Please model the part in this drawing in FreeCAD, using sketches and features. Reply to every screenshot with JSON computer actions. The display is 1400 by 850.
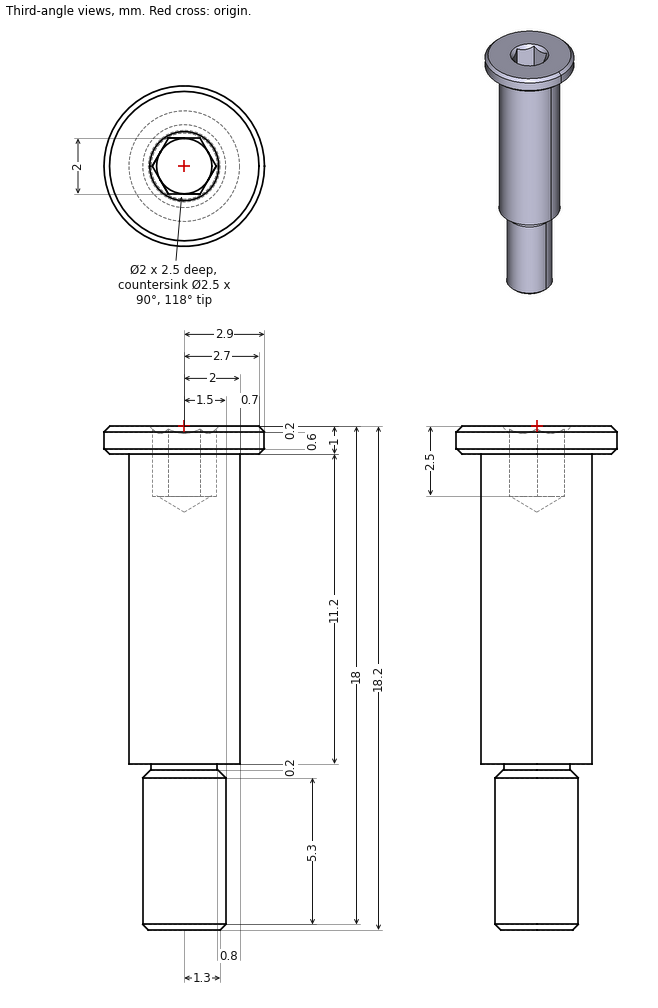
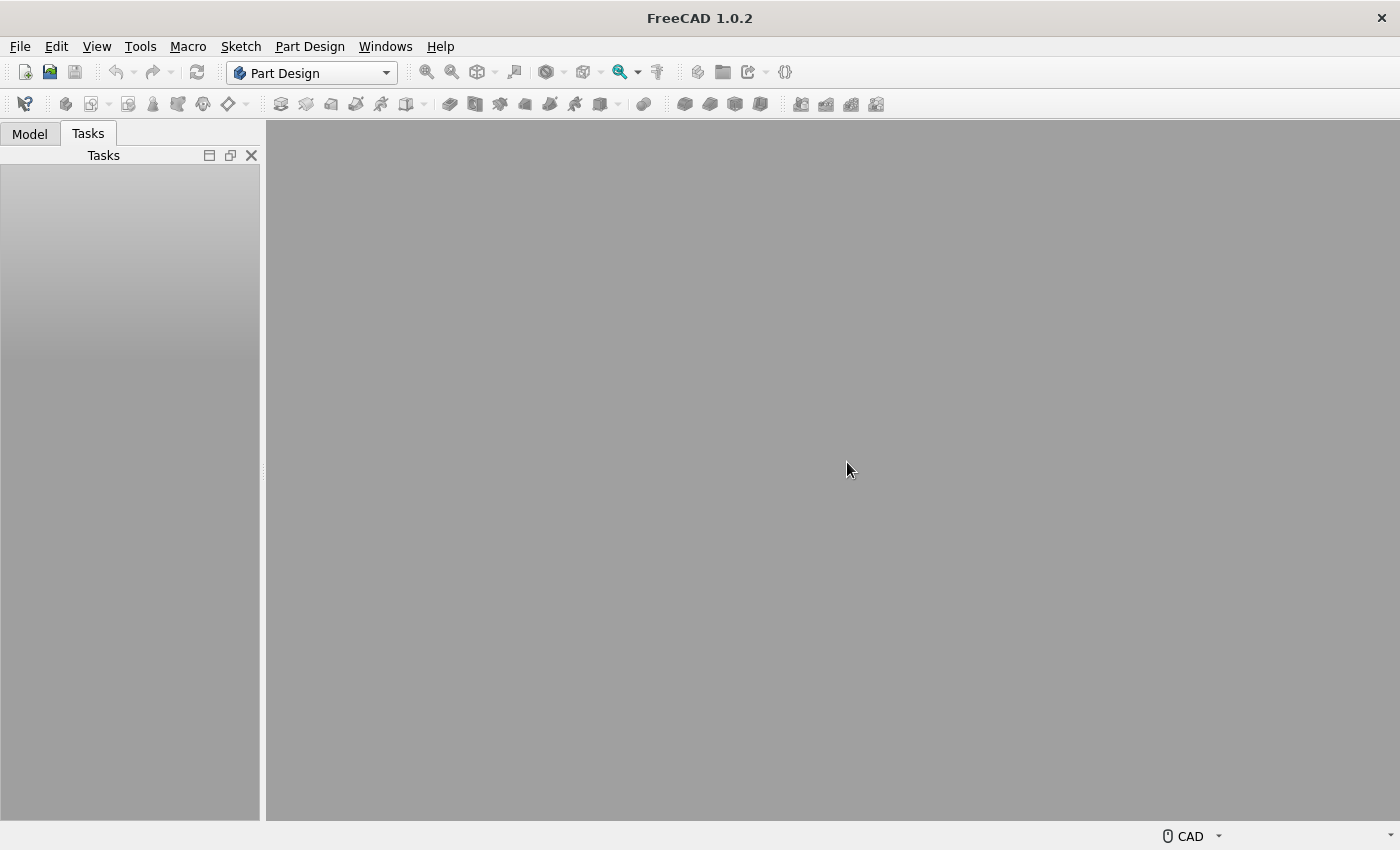
{"action": "left_click", "coordinate": [25, 72]}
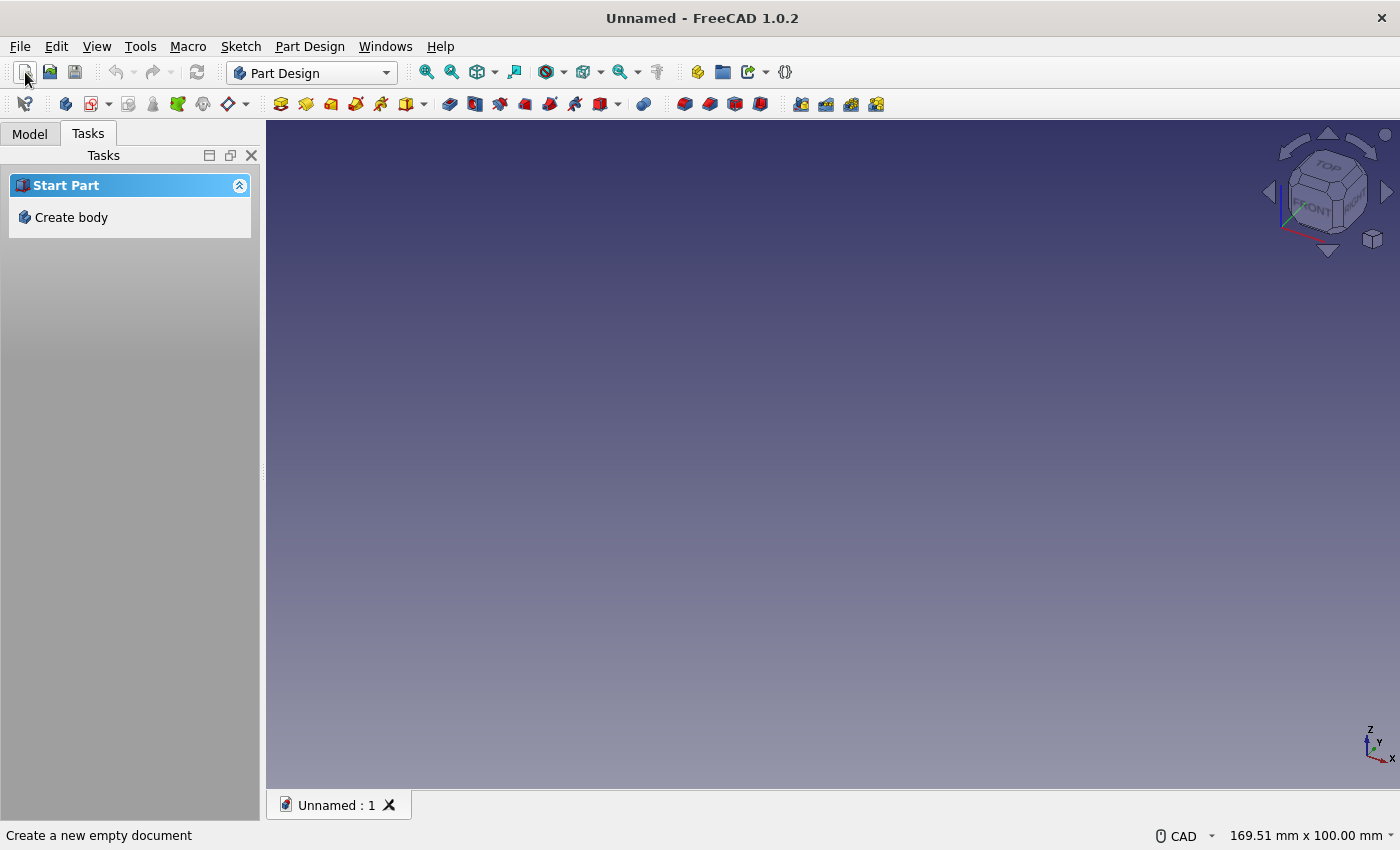
{"action": "left_click", "coordinate": [90, 104]}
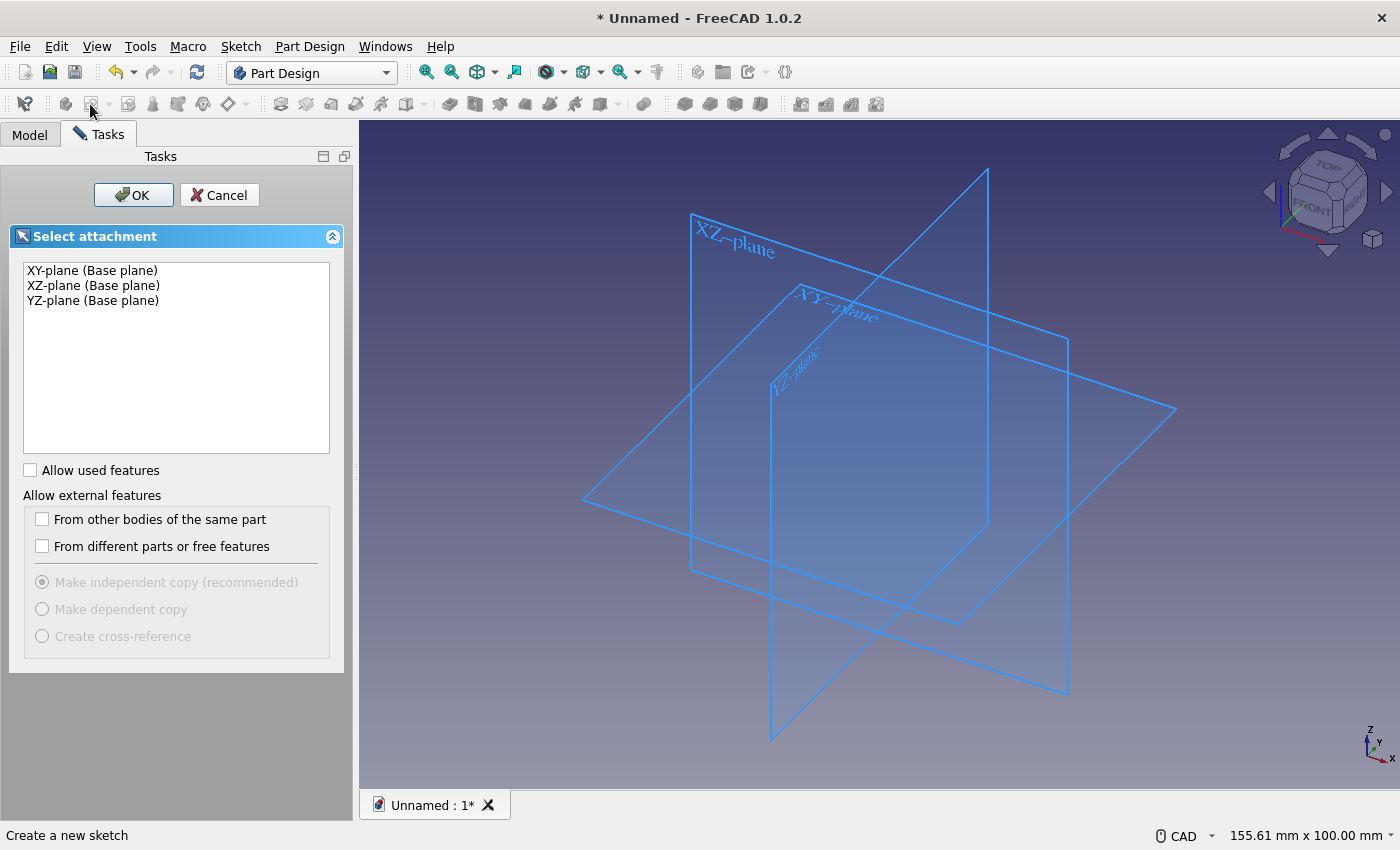
{"action": "left_click", "coordinate": [84, 286]}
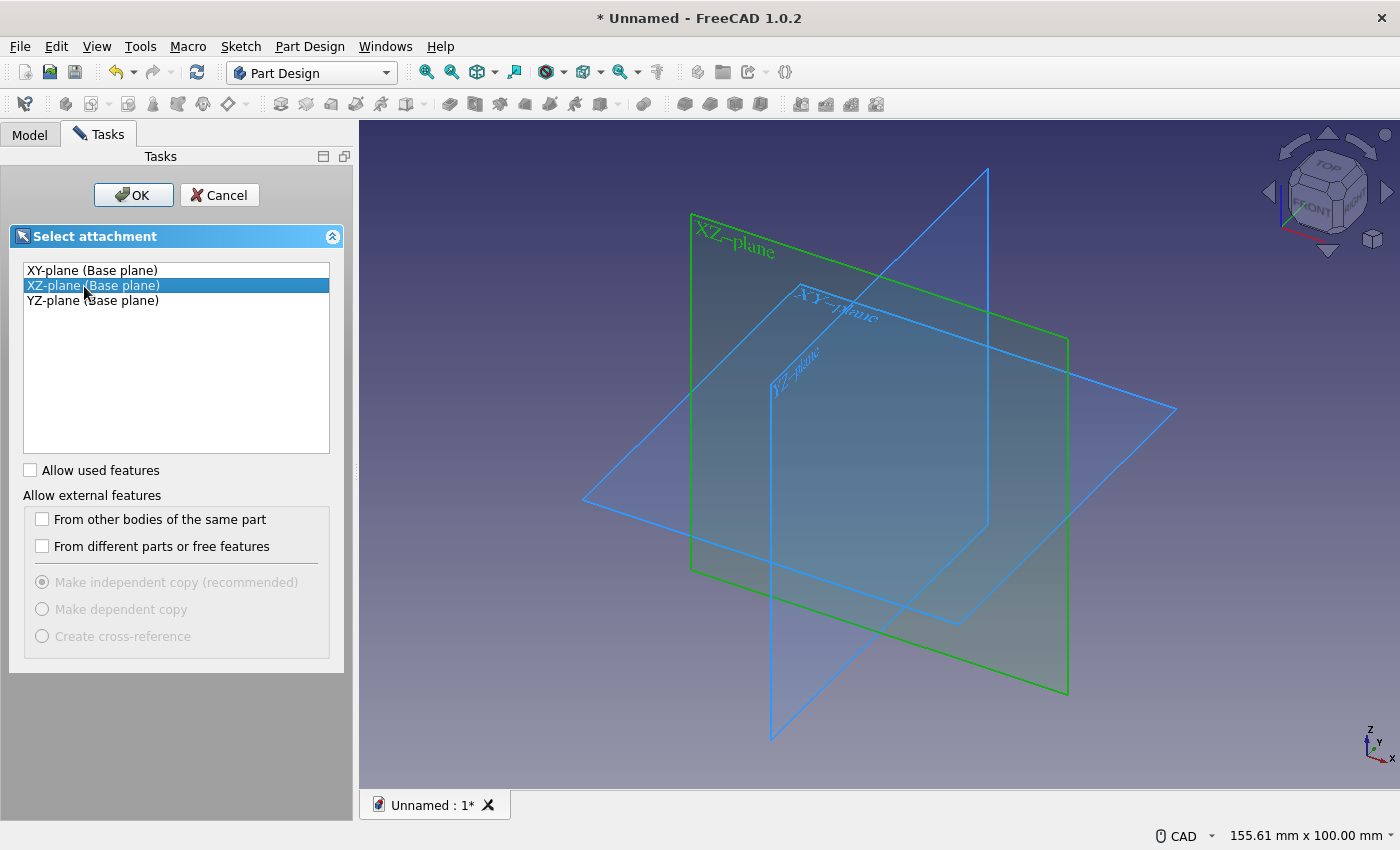
{"action": "left_click", "coordinate": [134, 195]}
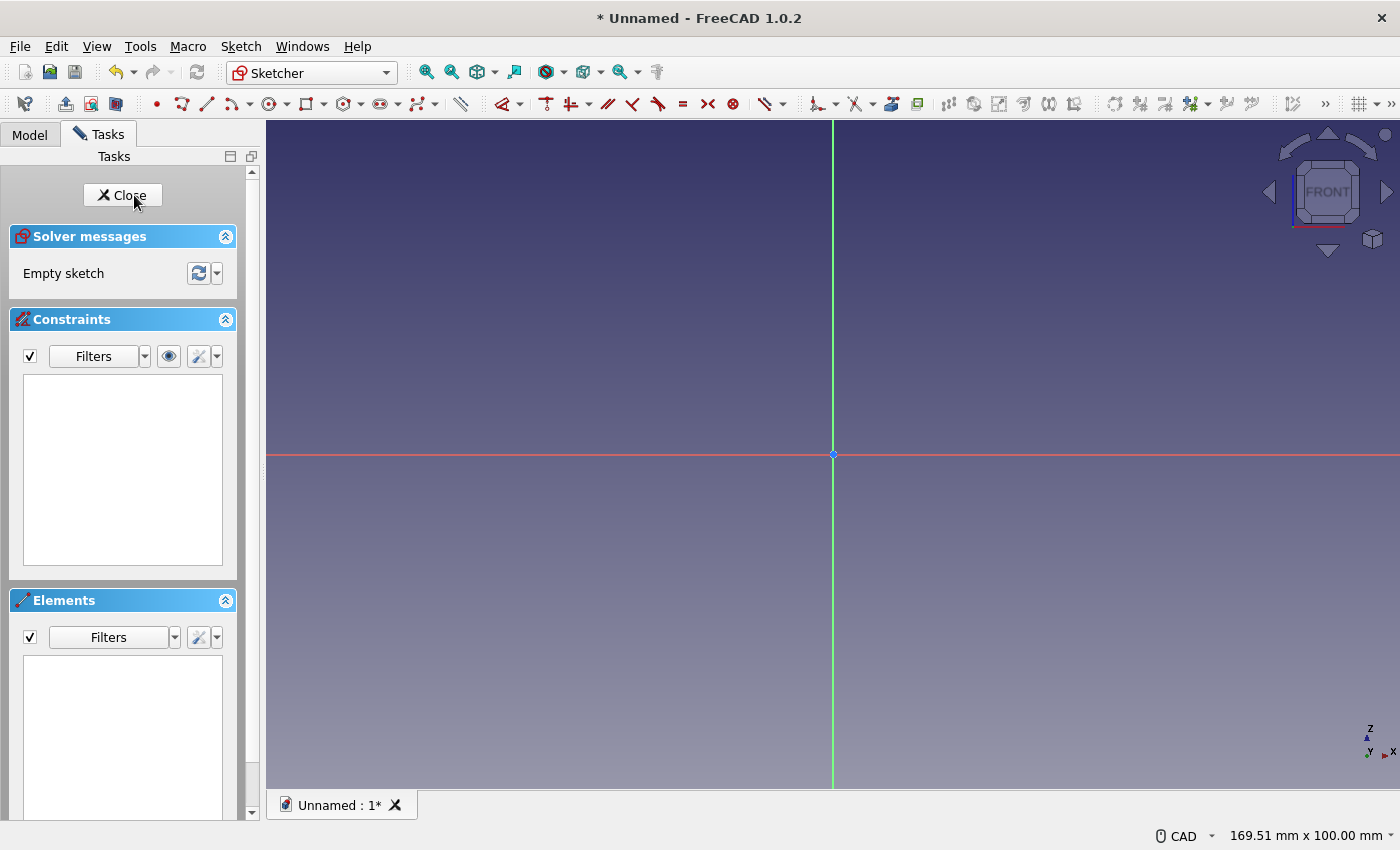
{"action": "scroll", "coordinate": [876, 542], "scroll_direction": "up", "scroll_amount": 6}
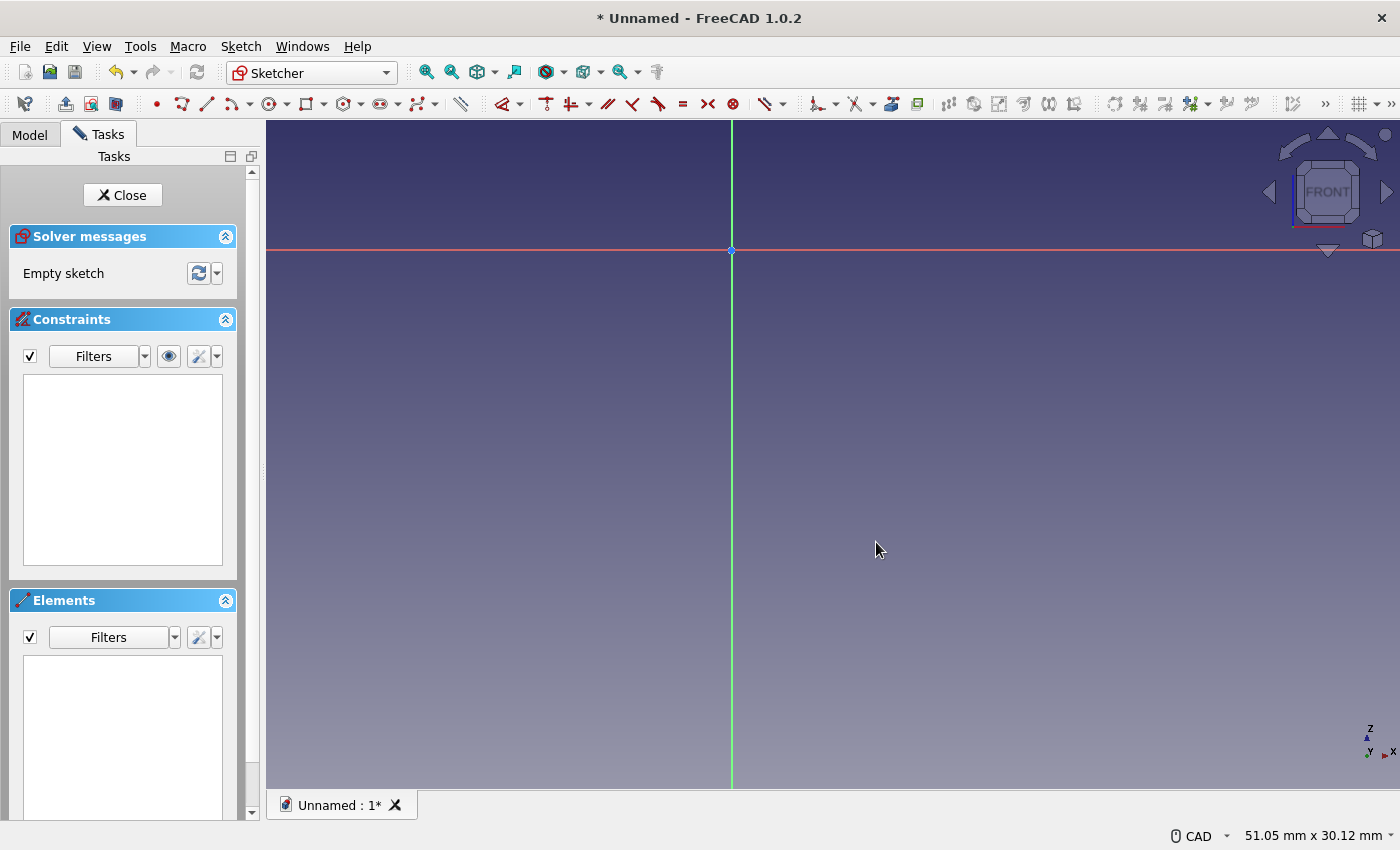
{"action": "left_click", "coordinate": [182, 104]}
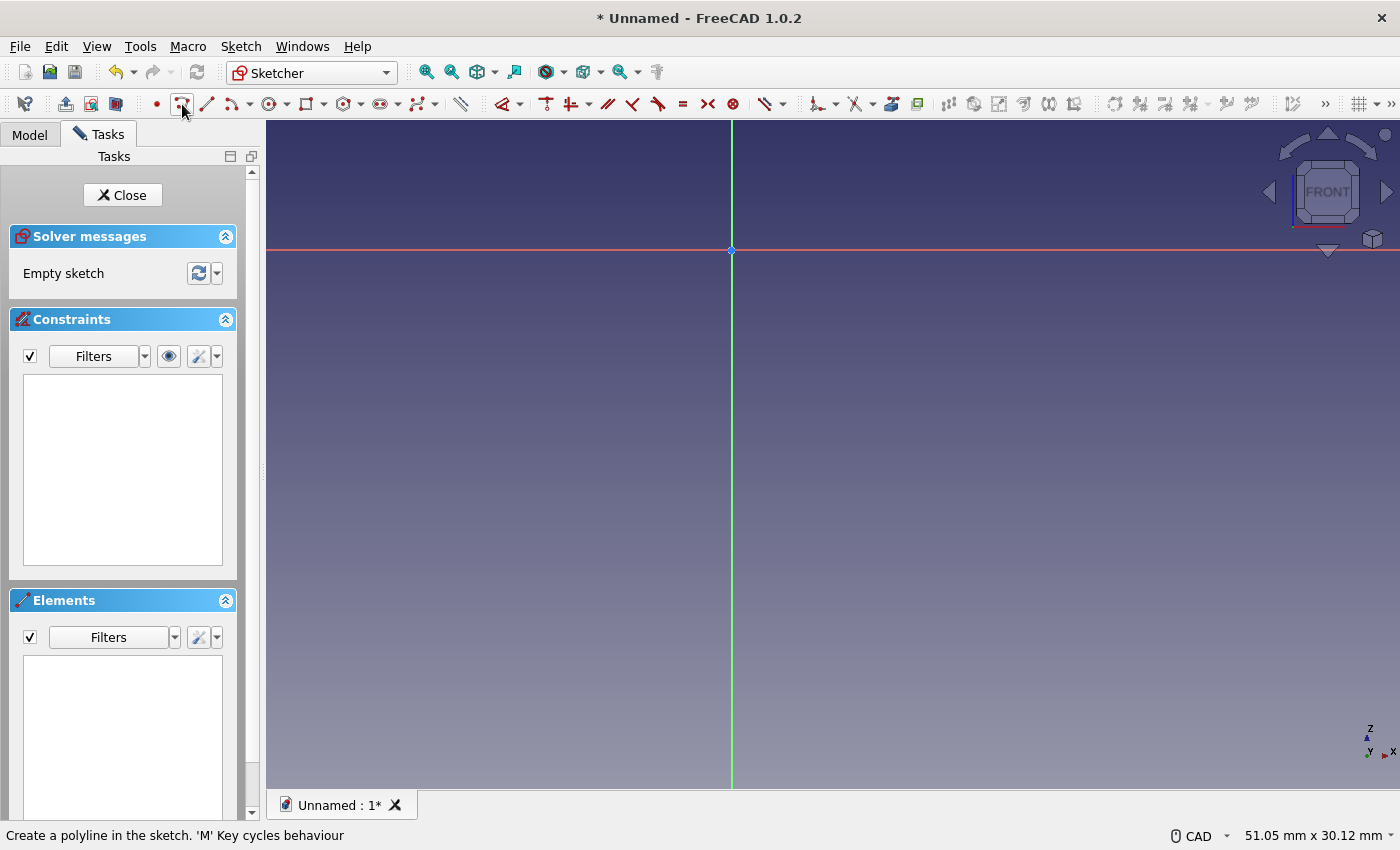
{"action": "left_click", "coordinate": [732, 250]}
{"action": "left_click", "coordinate": [792, 259]}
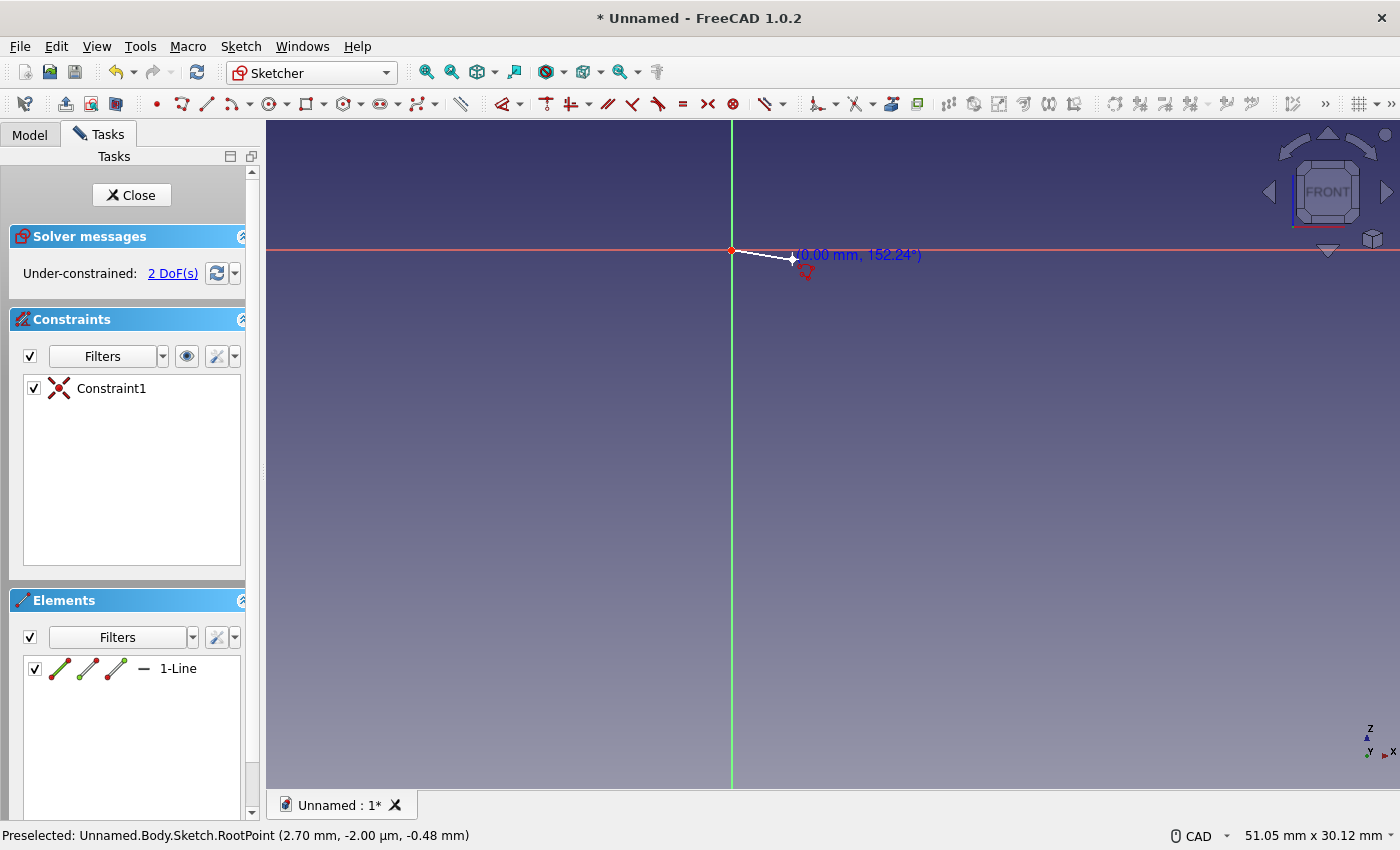
{"action": "scroll", "coordinate": [796, 254], "scroll_direction": "up", "scroll_amount": 7}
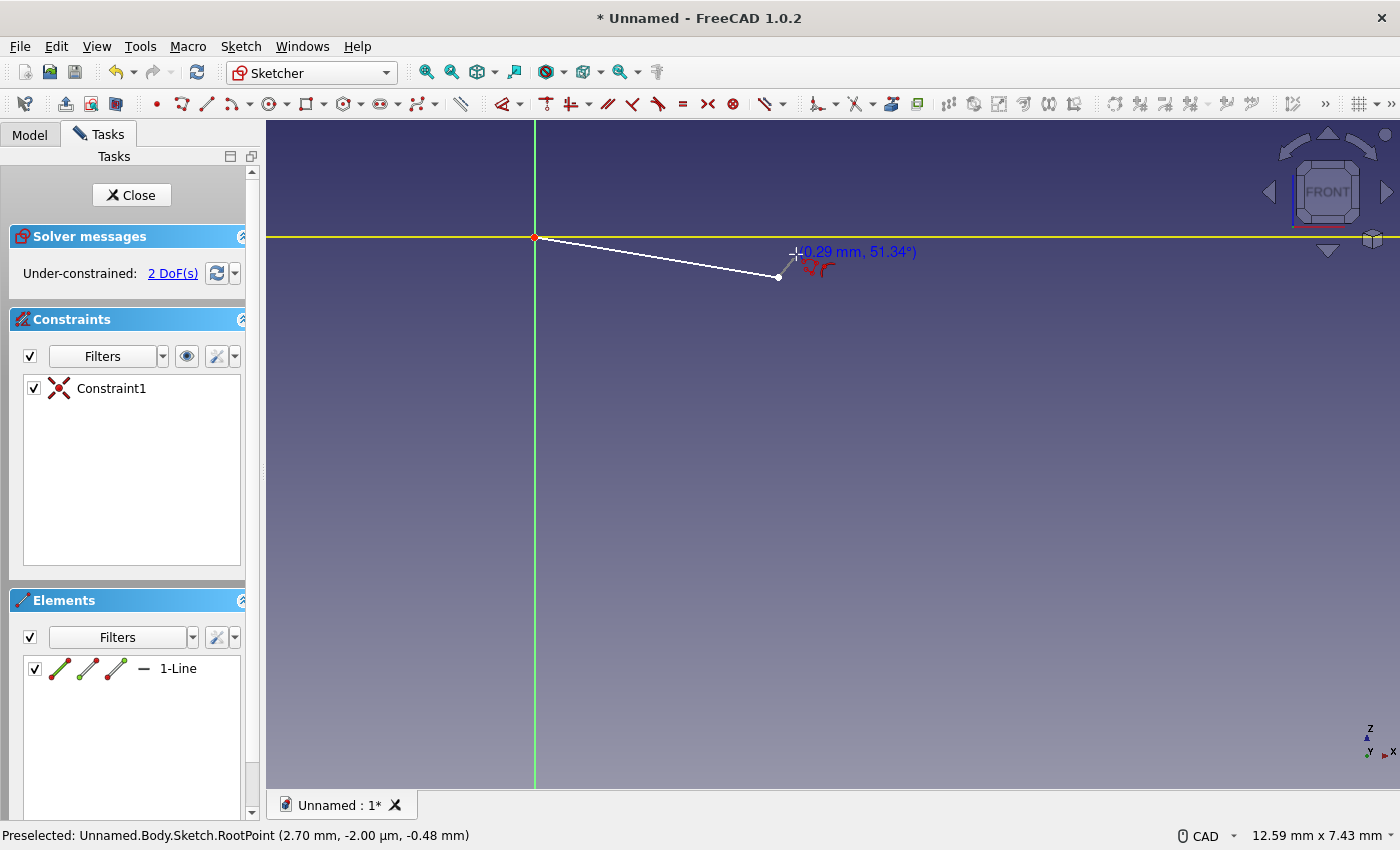
{"action": "left_click", "coordinate": [796, 255]}